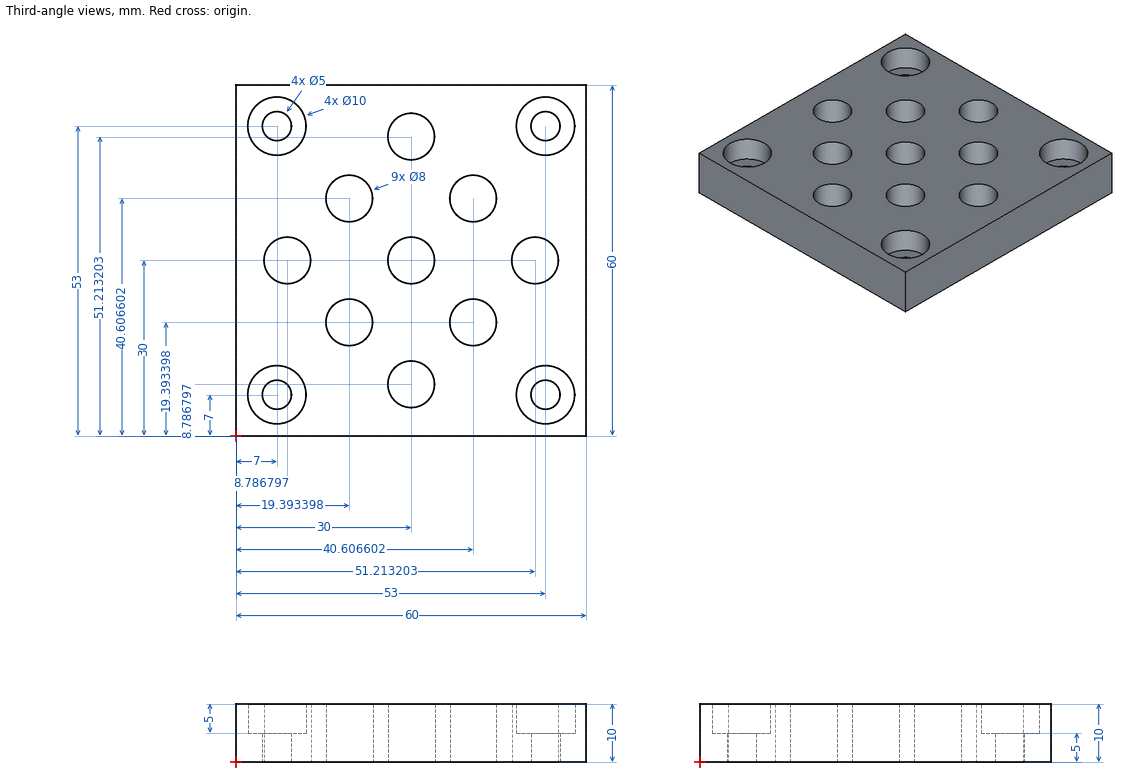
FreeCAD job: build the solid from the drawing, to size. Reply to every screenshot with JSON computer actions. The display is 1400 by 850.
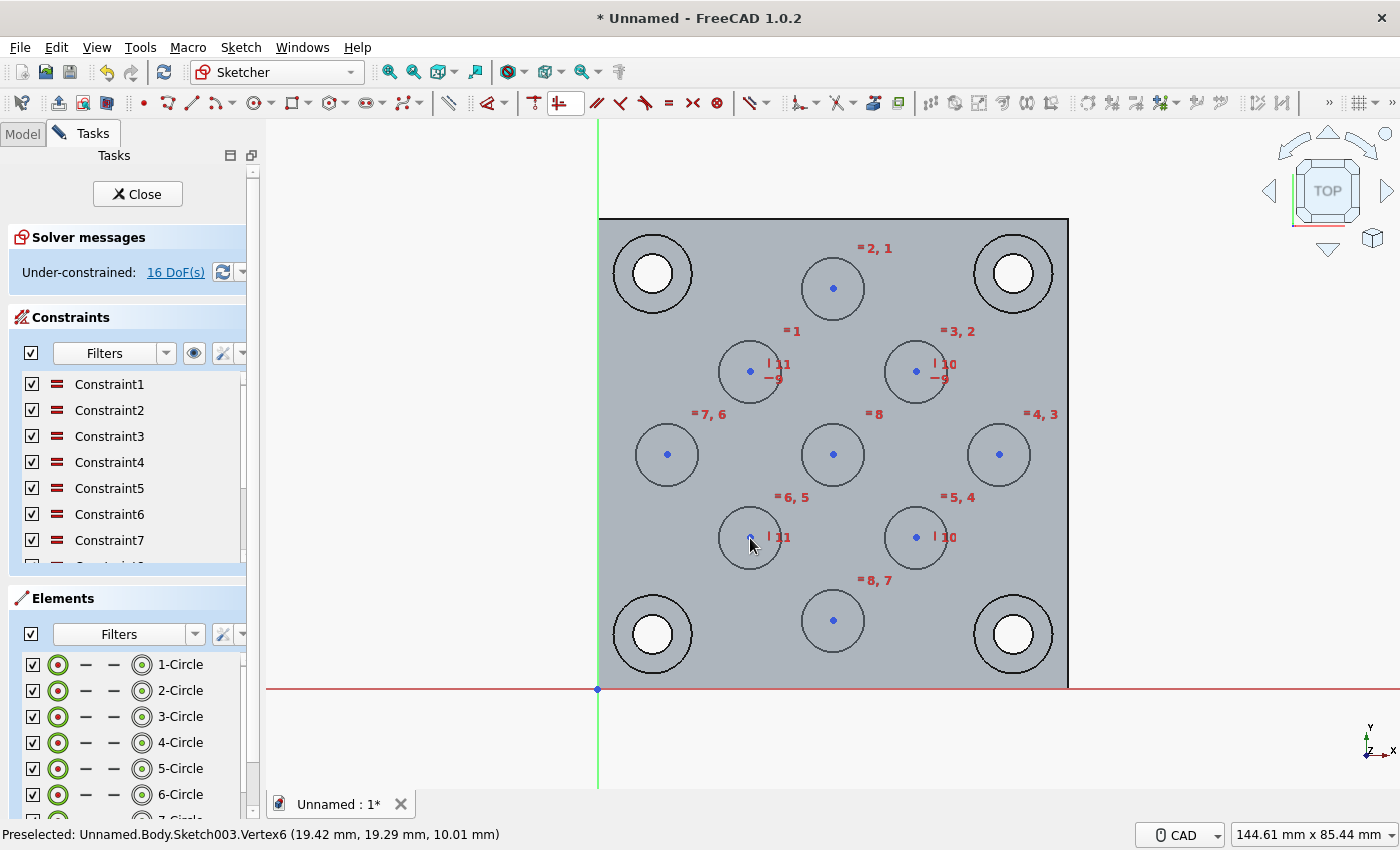
{"action": "left_click", "coordinate": [916, 538]}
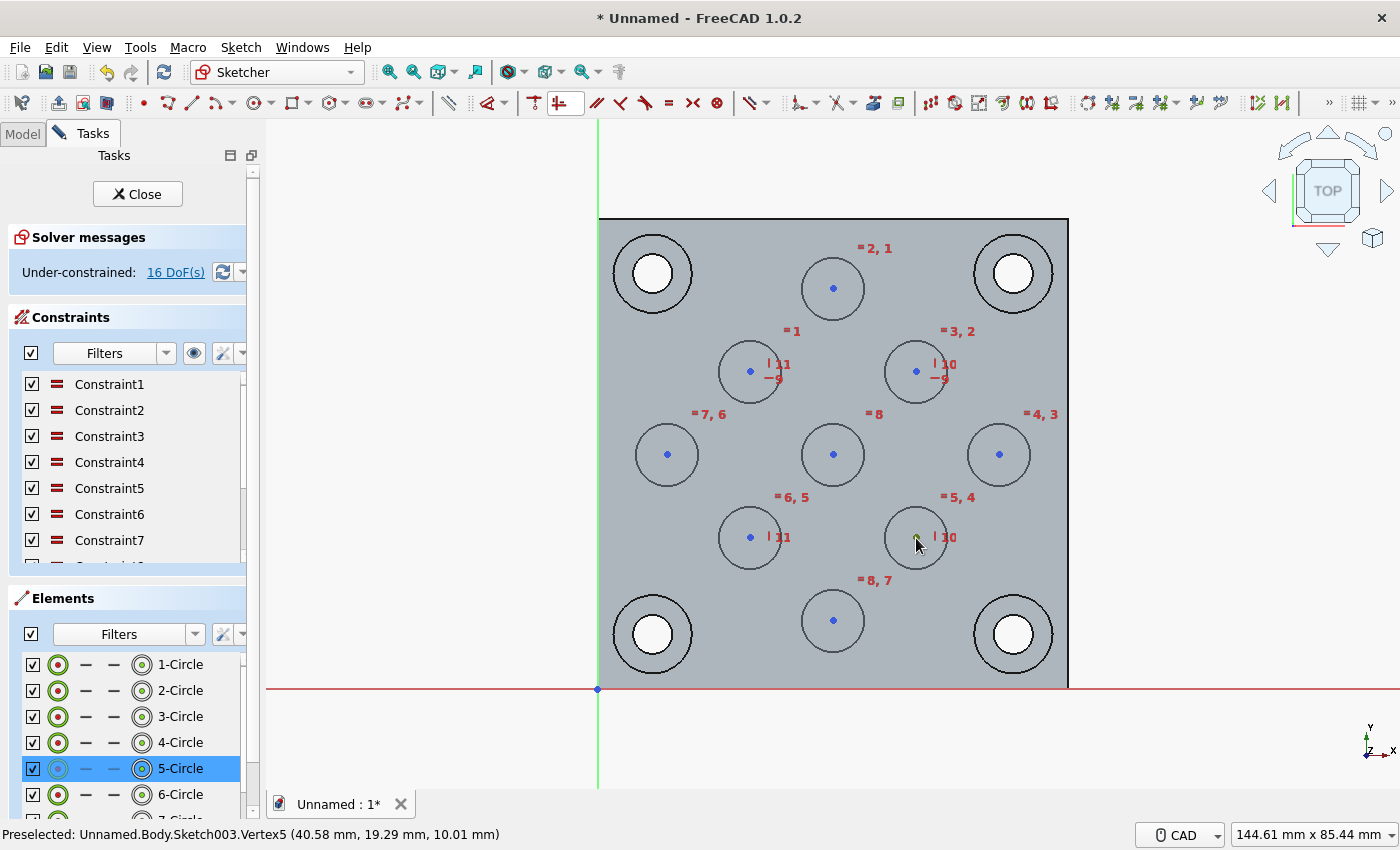
{"action": "left_click", "coordinate": [750, 538]}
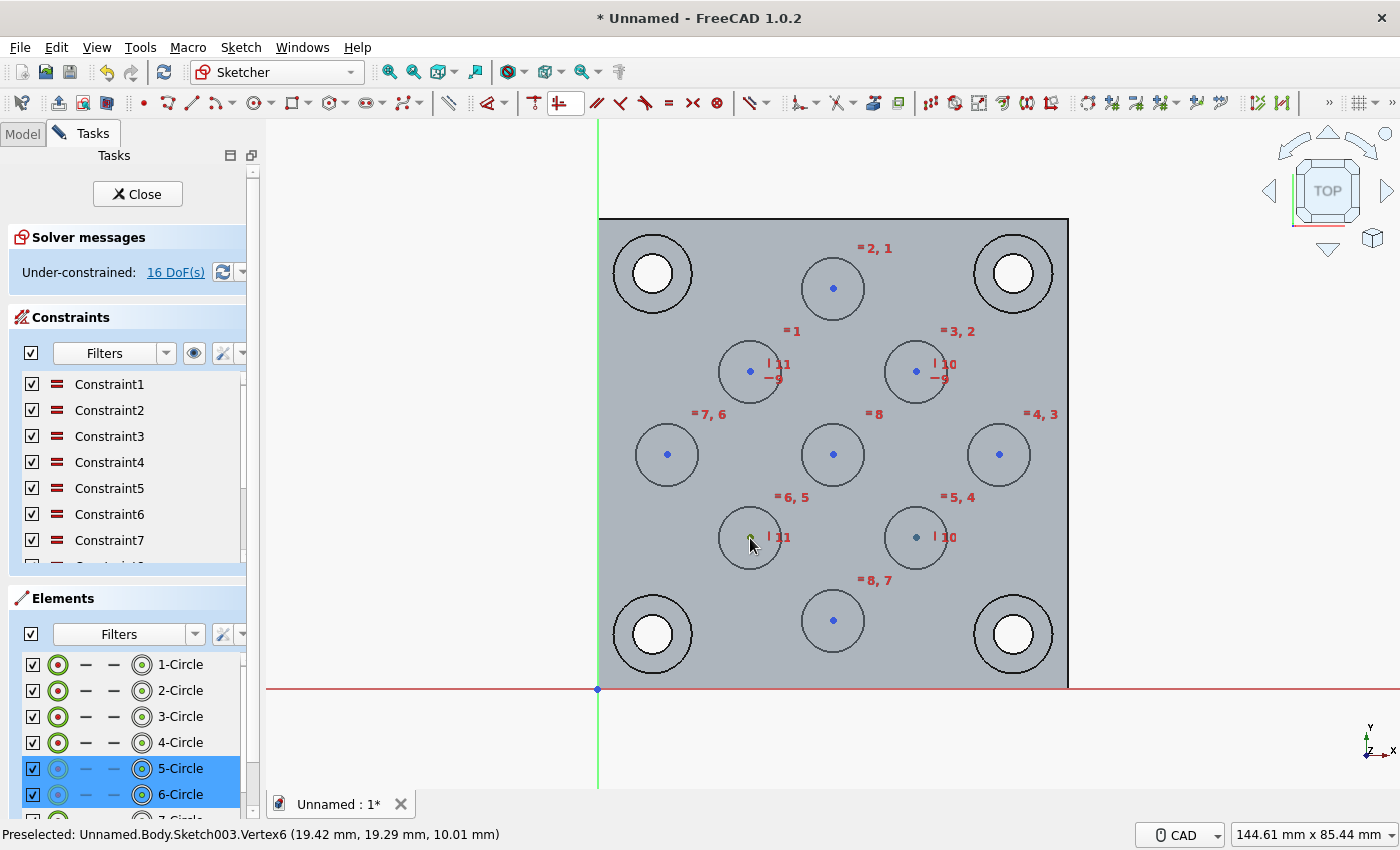
{"action": "left_click", "coordinate": [578, 104]}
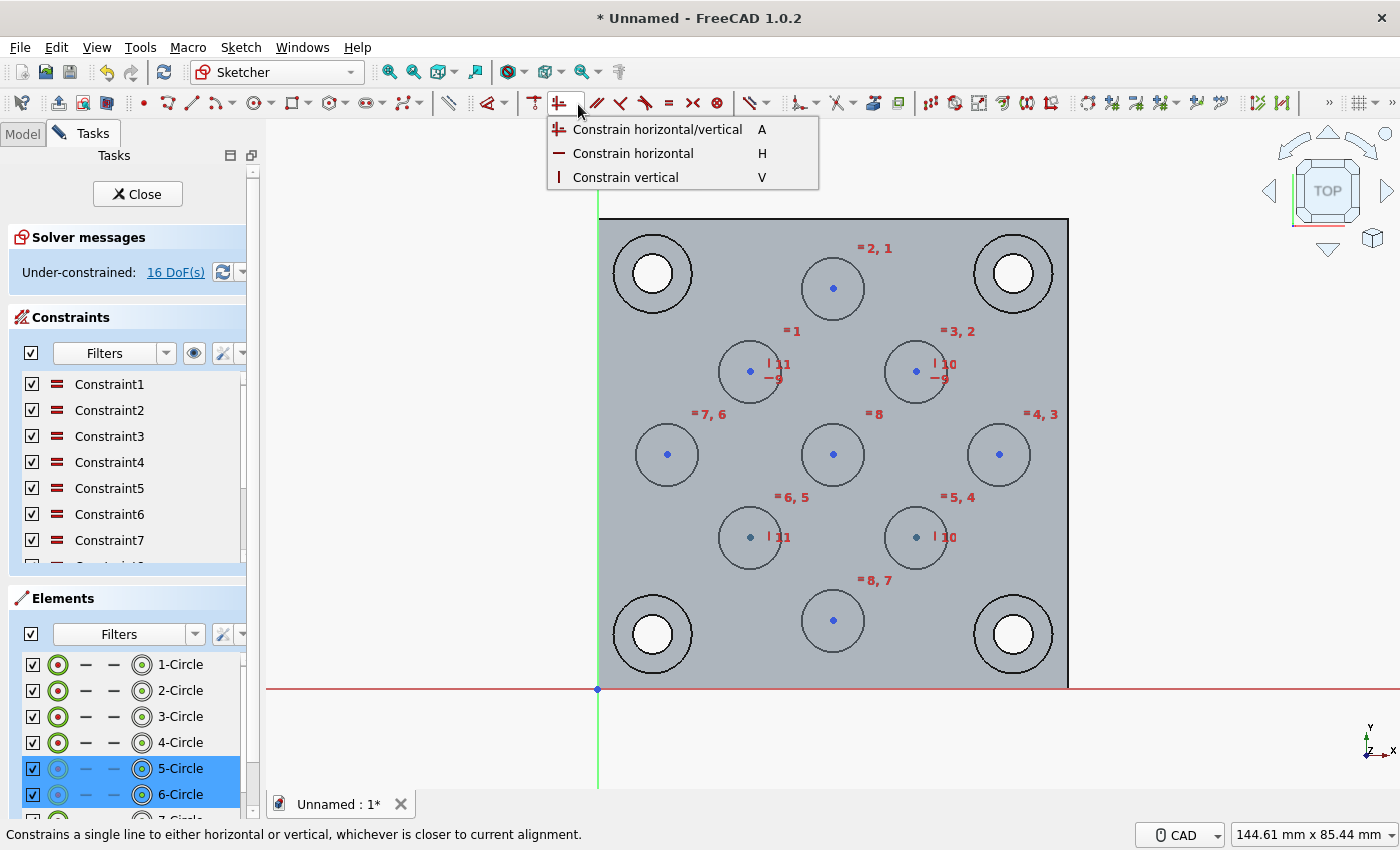
{"action": "left_click", "coordinate": [683, 153]}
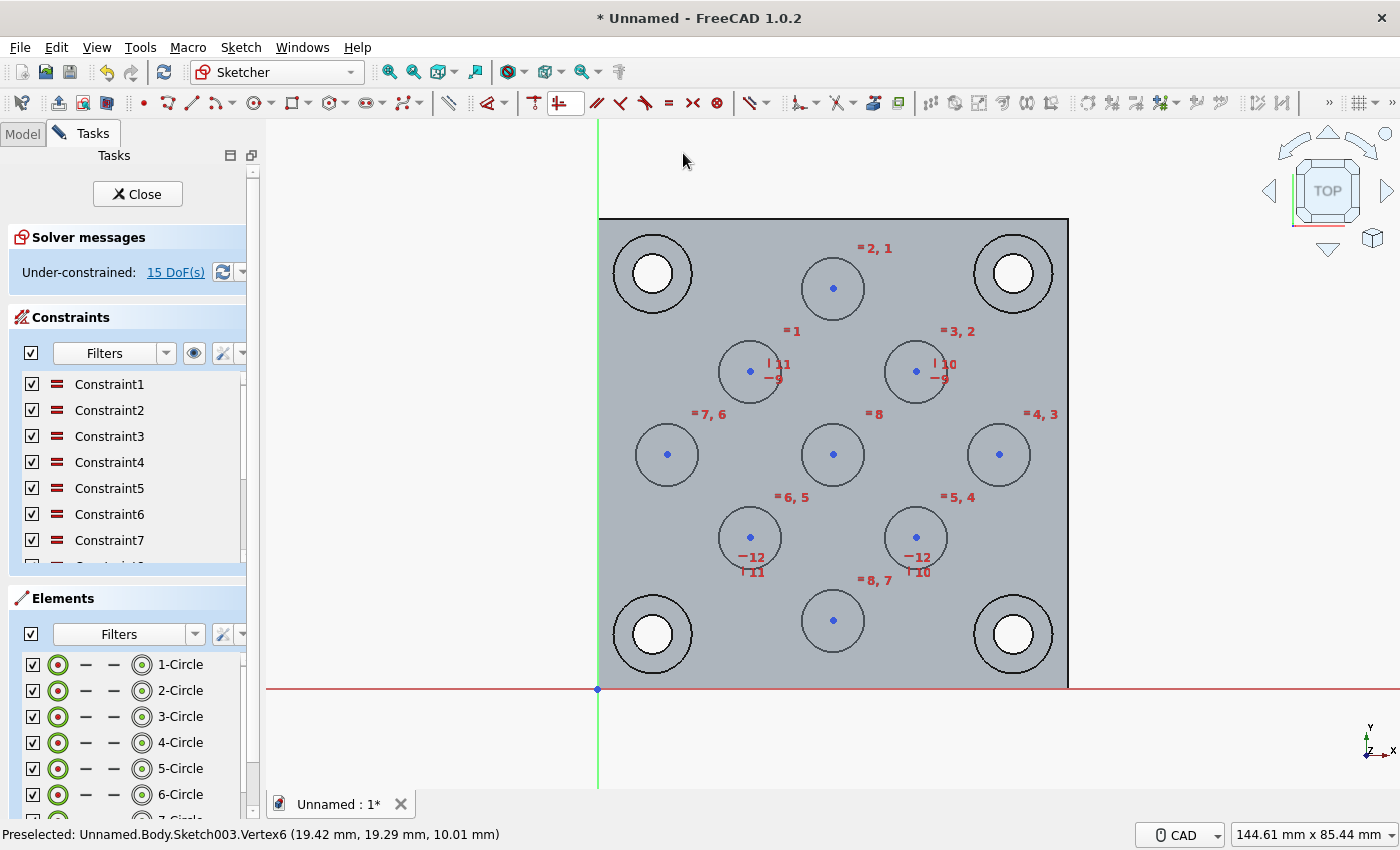
{"action": "left_click", "coordinate": [999, 455]}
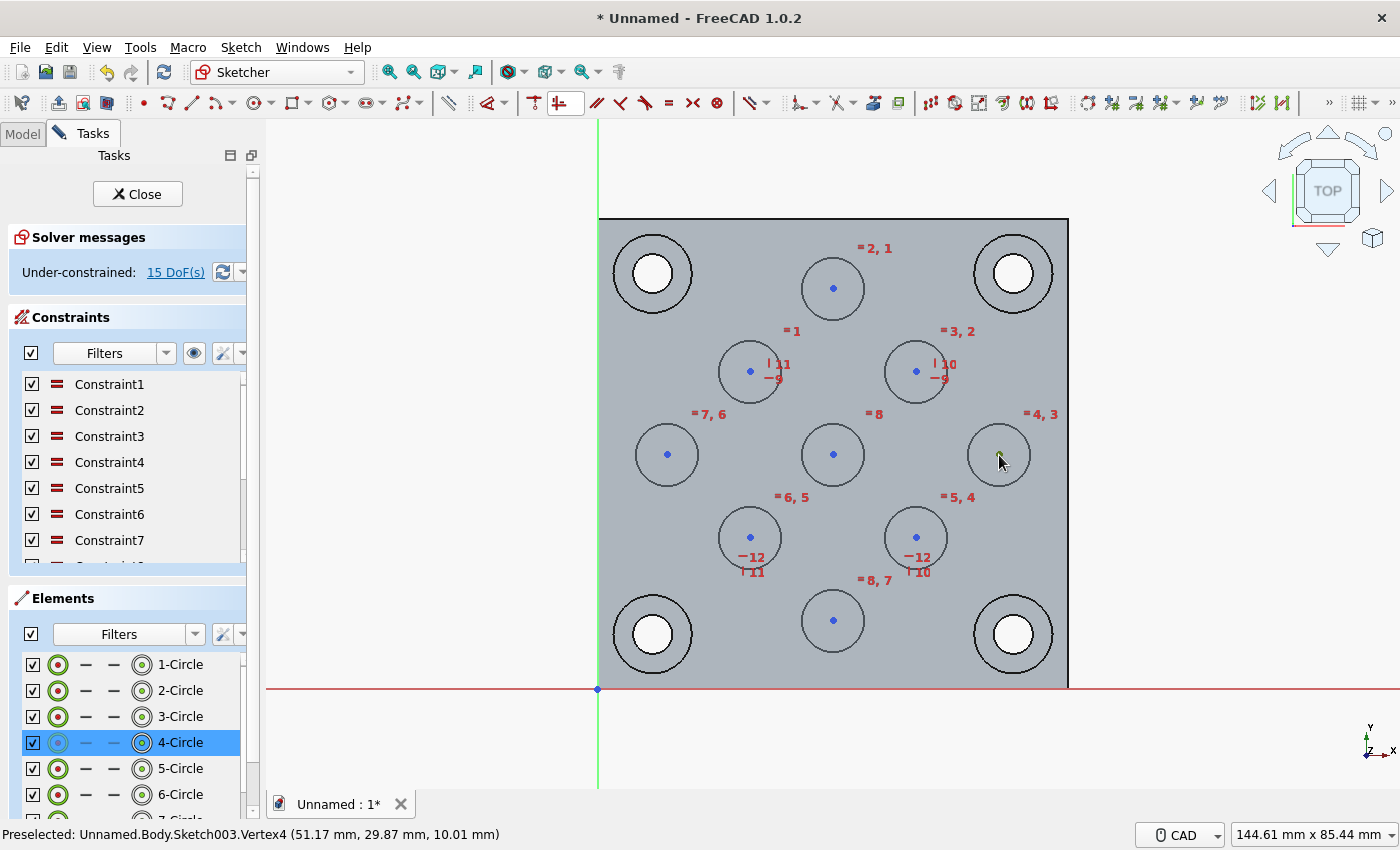
{"action": "left_click", "coordinate": [667, 455]}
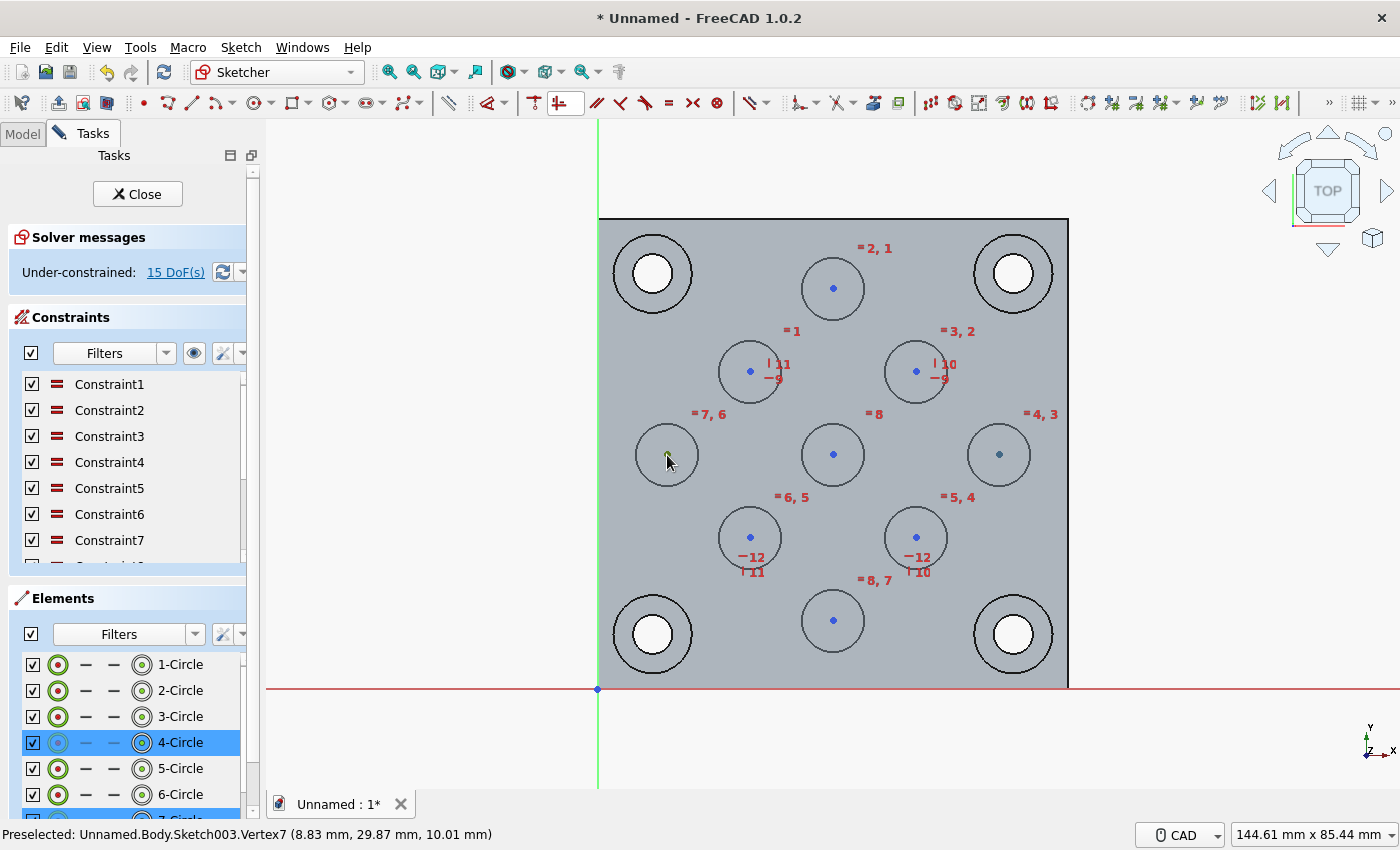
{"action": "key", "text": "h"}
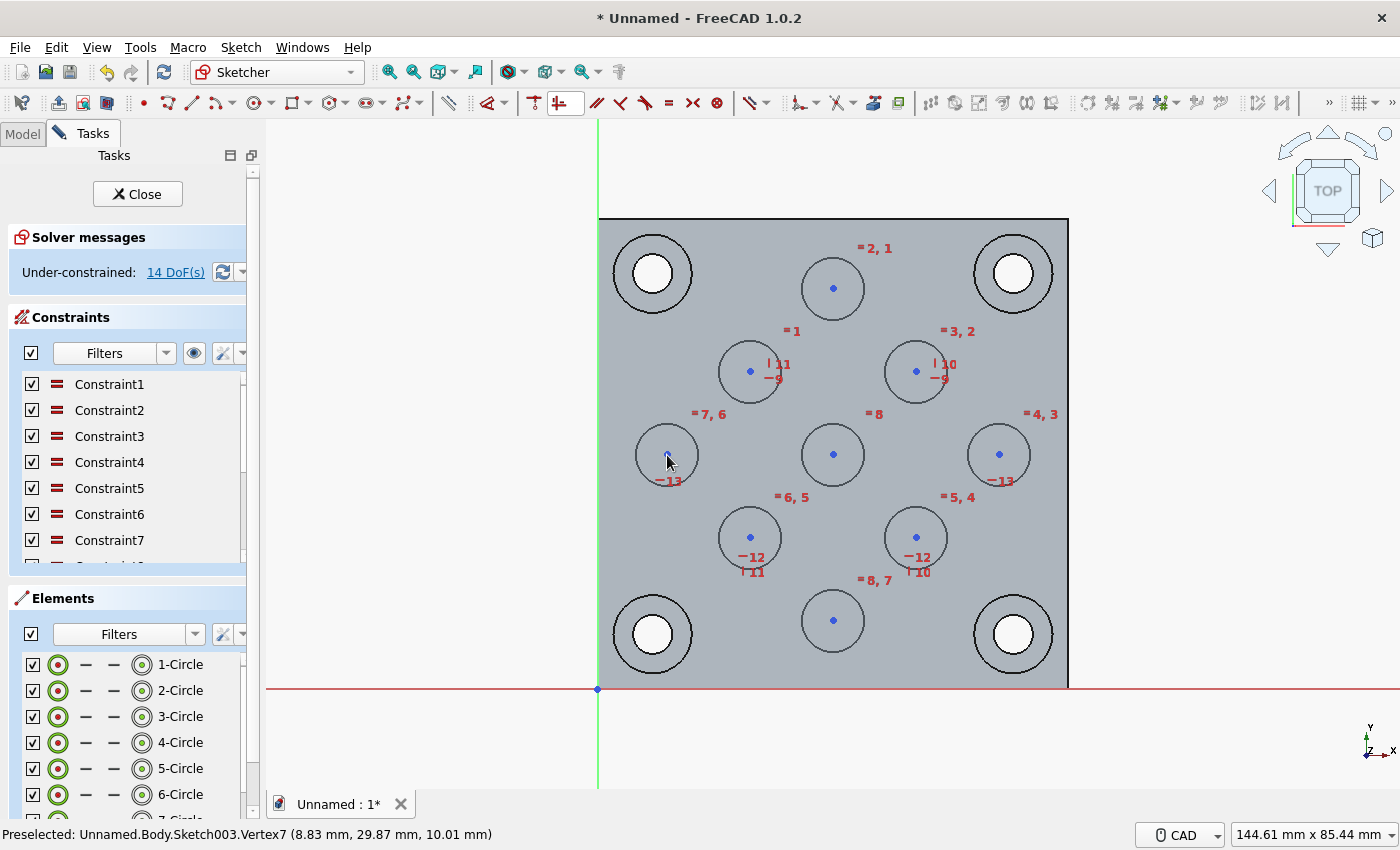
{"action": "left_click", "coordinate": [833, 621]}